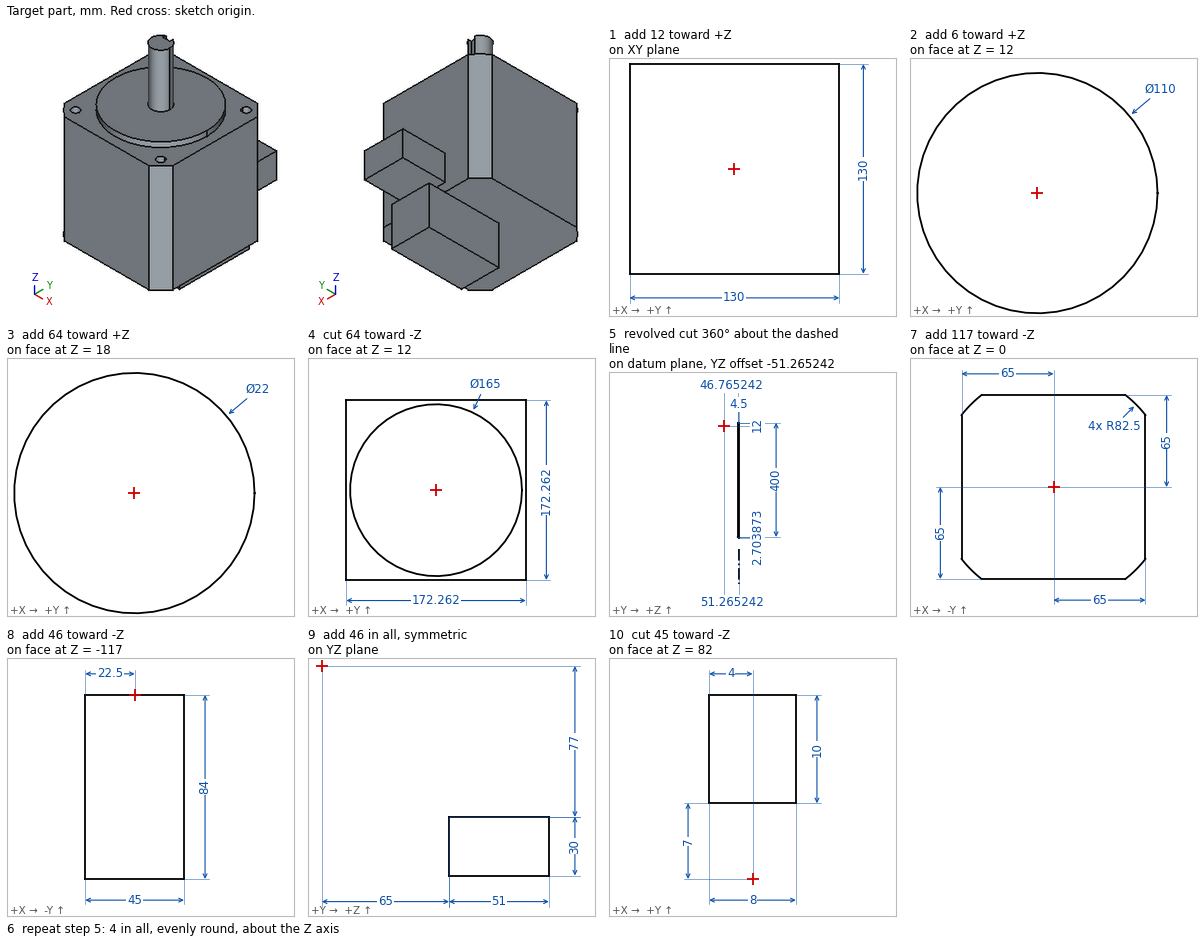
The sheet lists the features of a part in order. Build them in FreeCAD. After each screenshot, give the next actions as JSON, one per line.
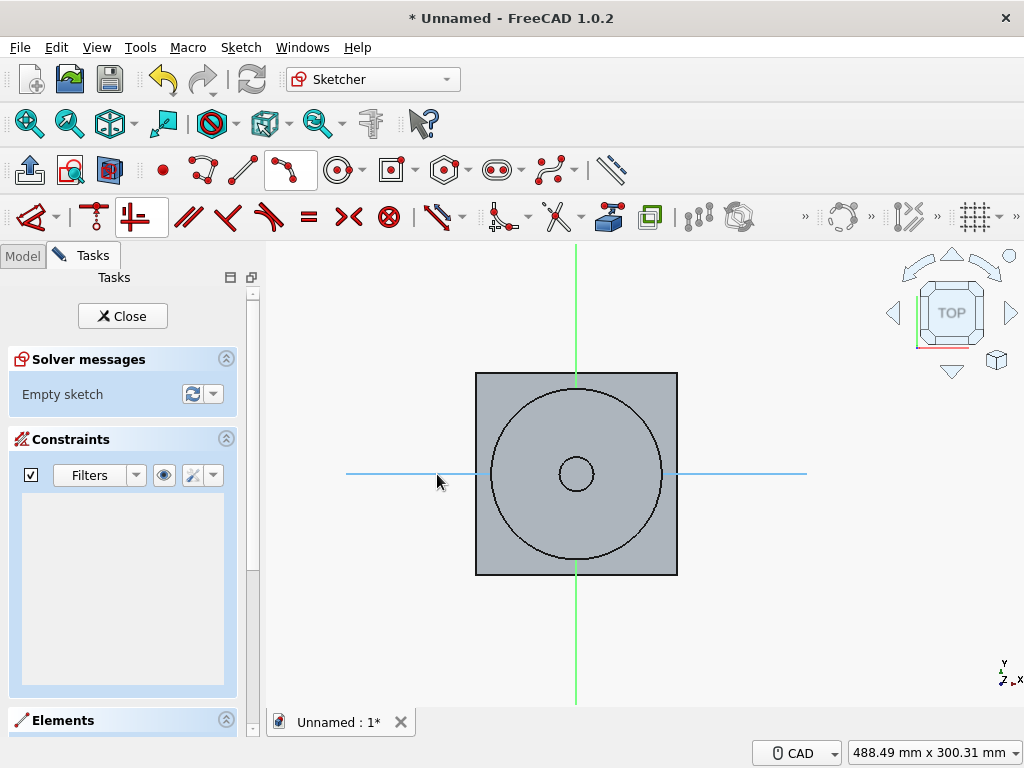
{"action": "left_click", "coordinate": [392, 170]}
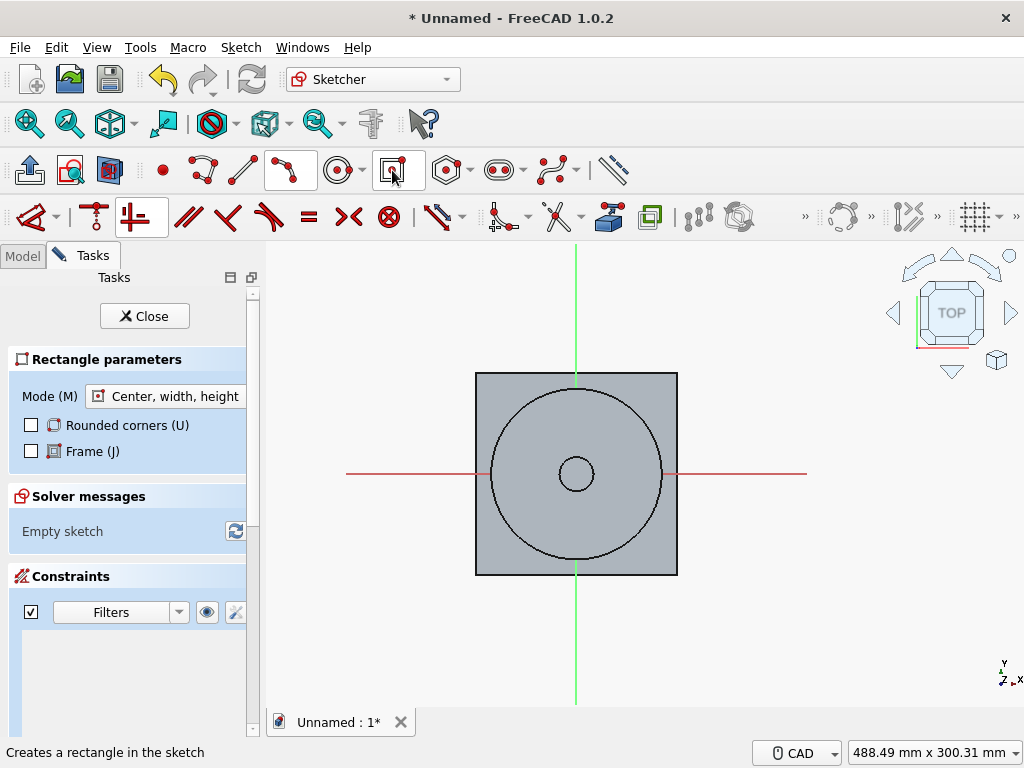
{"action": "left_click", "coordinate": [577, 474]}
{"action": "mouse_move", "coordinate": [710, 341]}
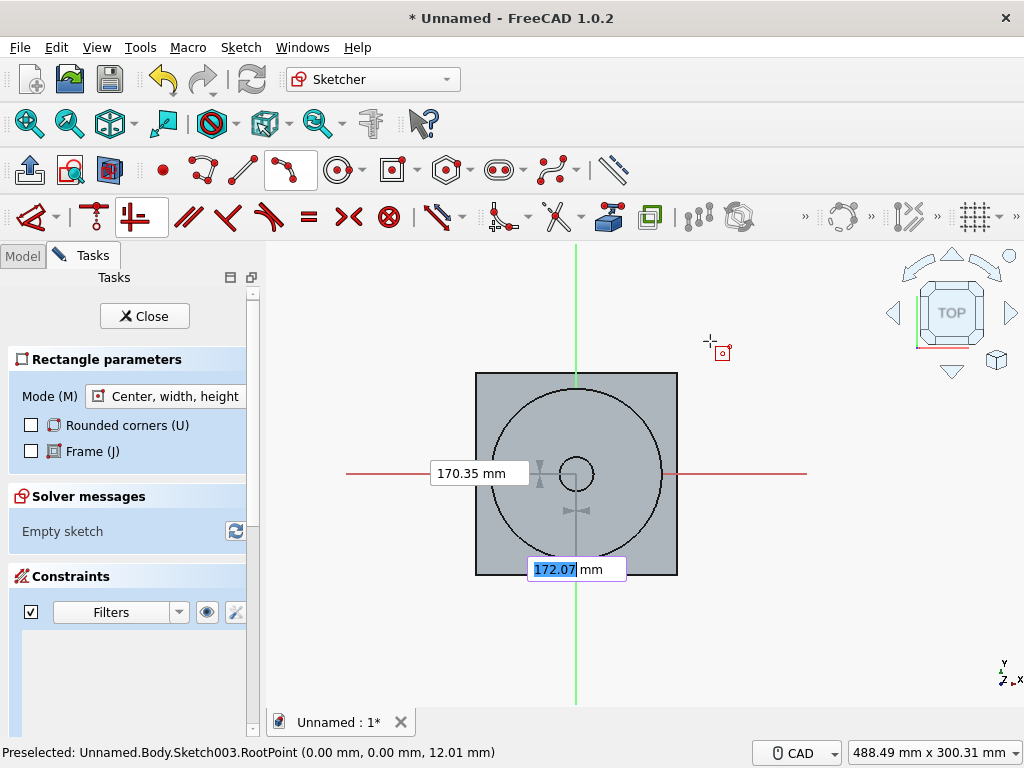
{"action": "type", "text": "172.262"}
{"action": "key", "text": "Tab"}
{"action": "type", "text": "172.262"}
{"action": "key", "text": "Return"}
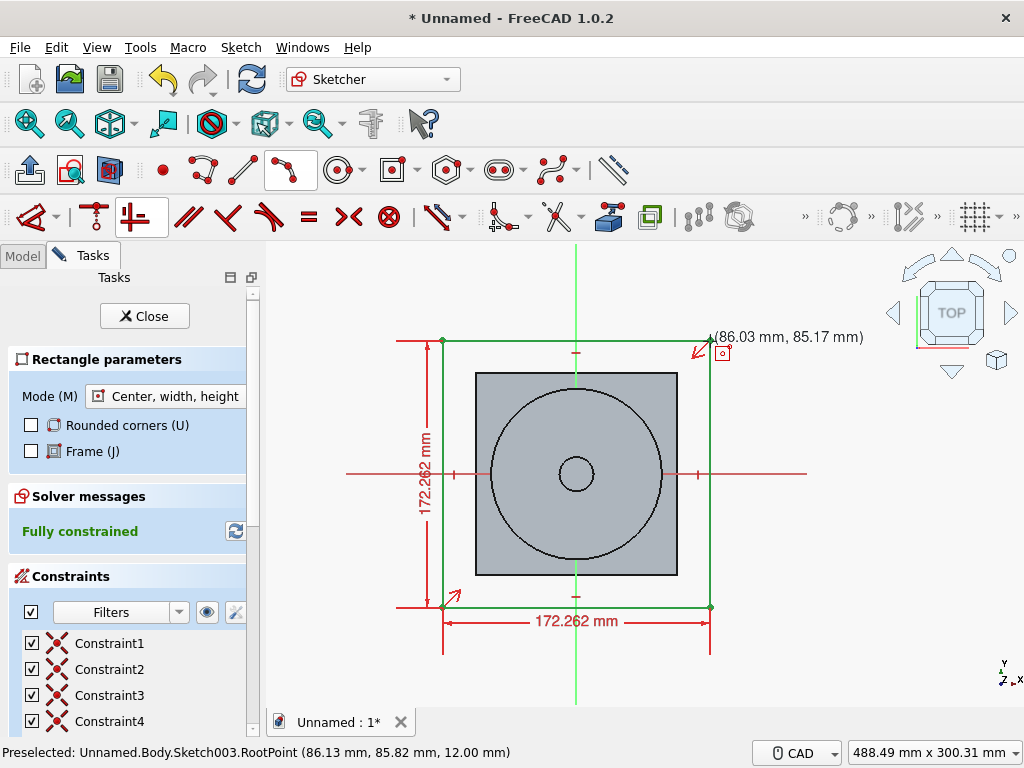
{"action": "left_click", "coordinate": [338, 170]}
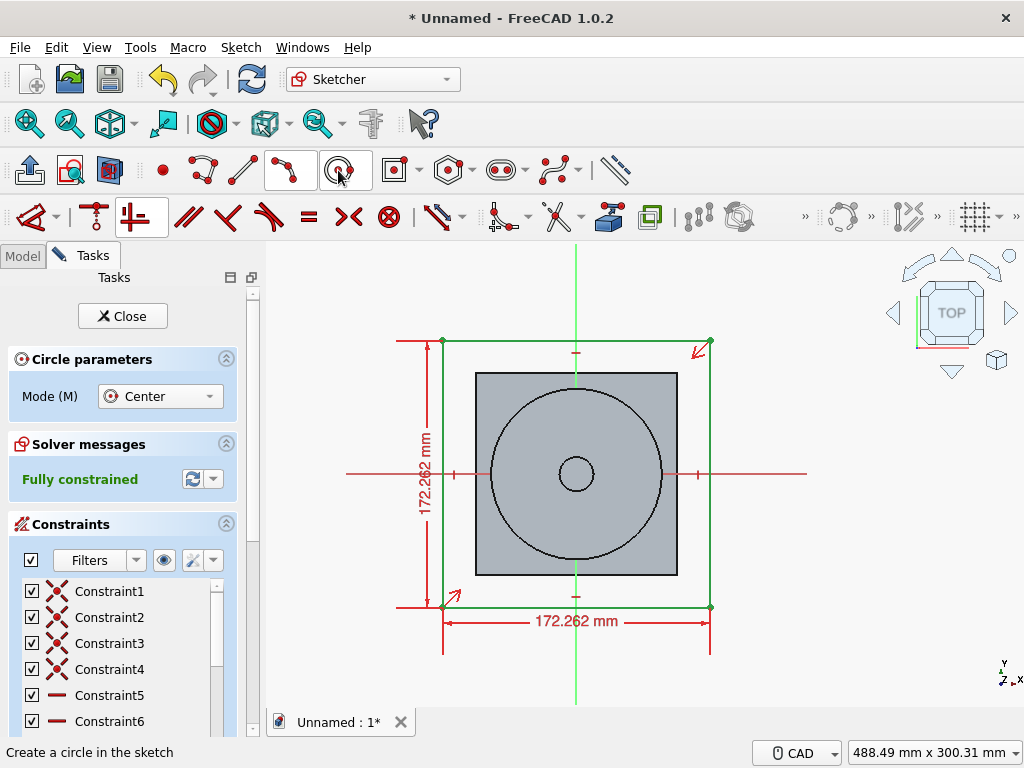
{"action": "left_click", "coordinate": [577, 474]}
{"action": "mouse_move", "coordinate": [667, 384]}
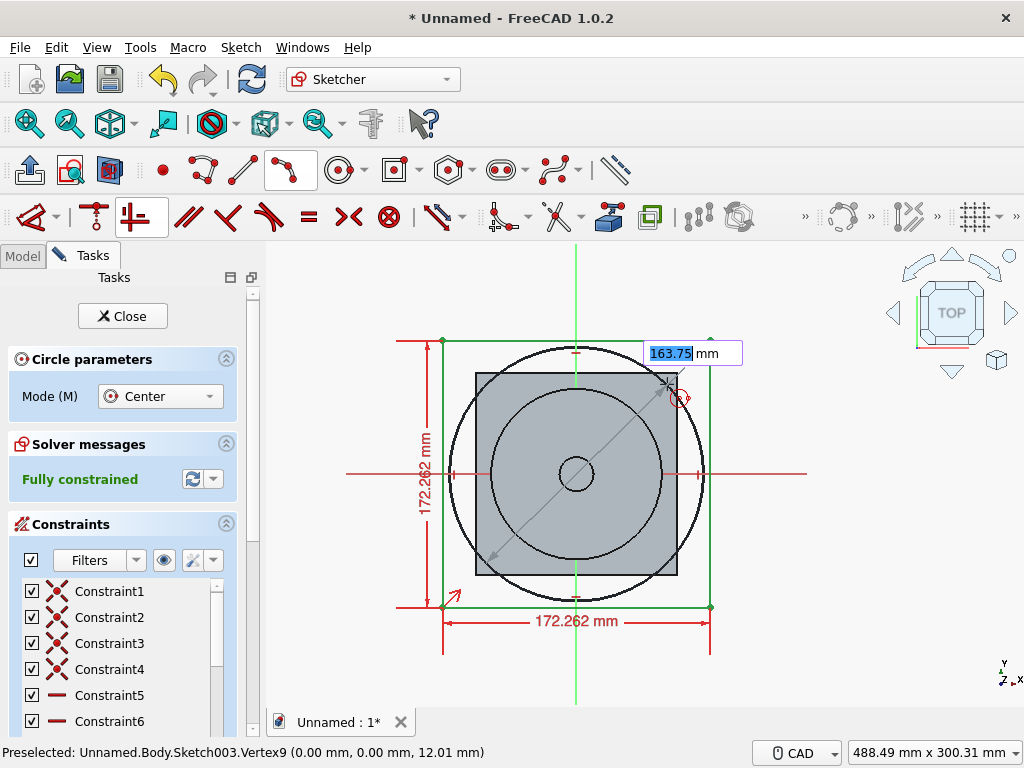
{"action": "type", "text": "165"}
{"action": "key", "text": "Return"}
{"action": "key", "text": "Escape"}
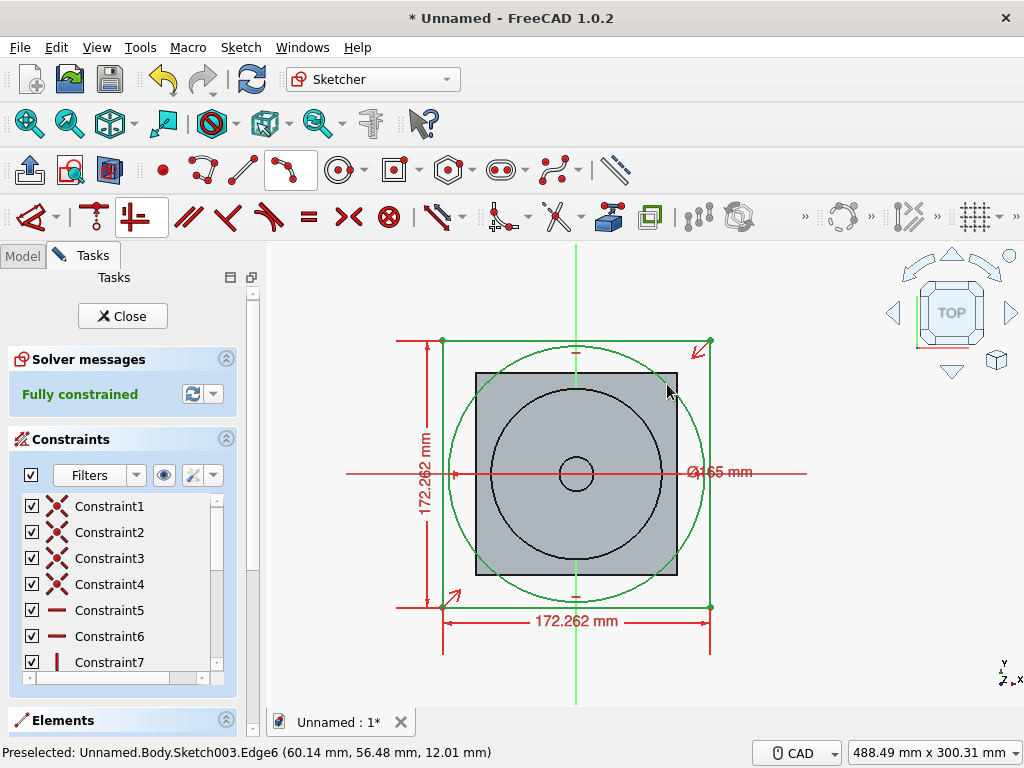
{"action": "left_click", "coordinate": [123, 316]}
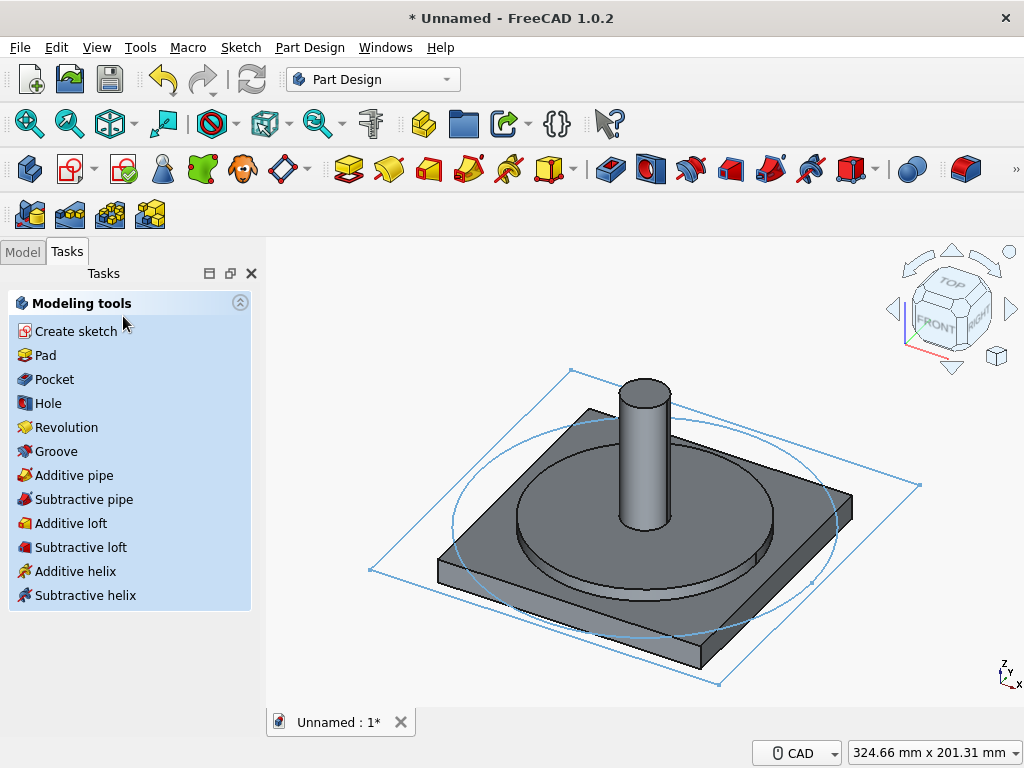
{"action": "left_click", "coordinate": [612, 170]}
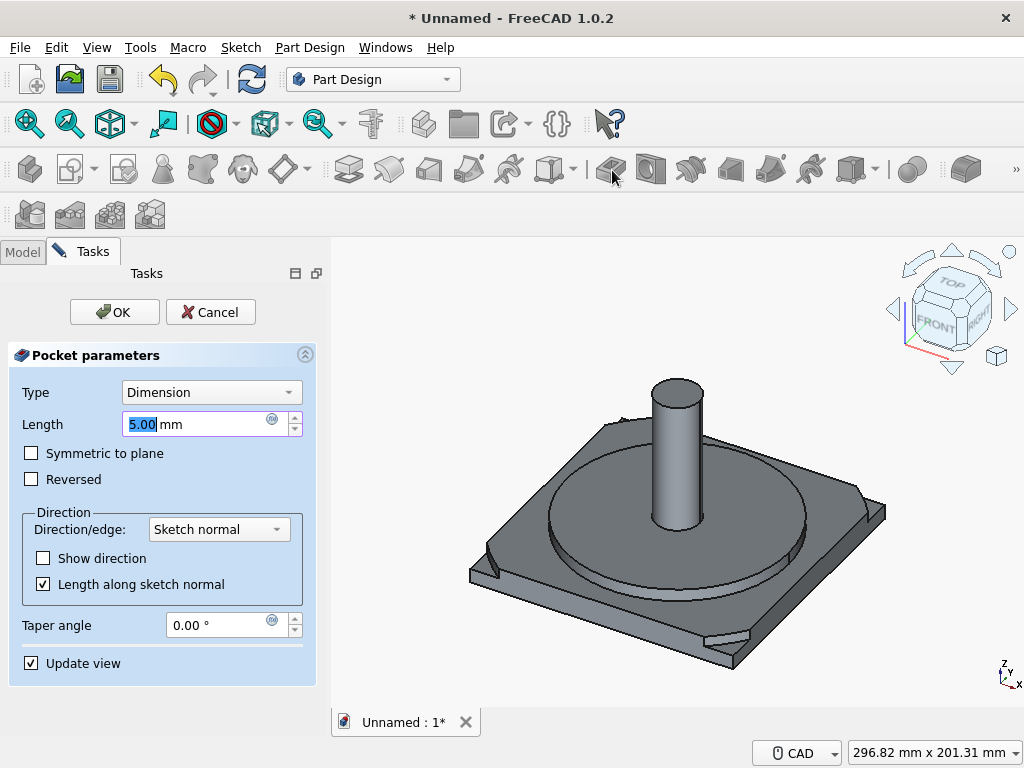
{"action": "type", "text": "64"}
{"action": "key", "text": "Tab"}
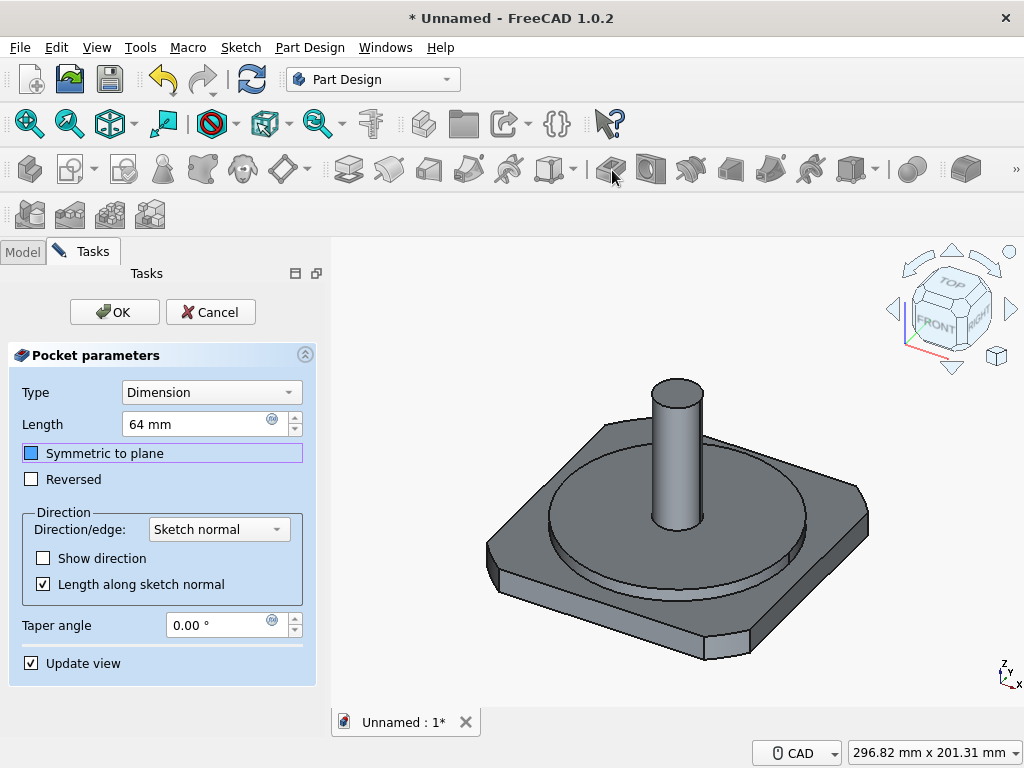
{"action": "left_click", "coordinate": [115, 312]}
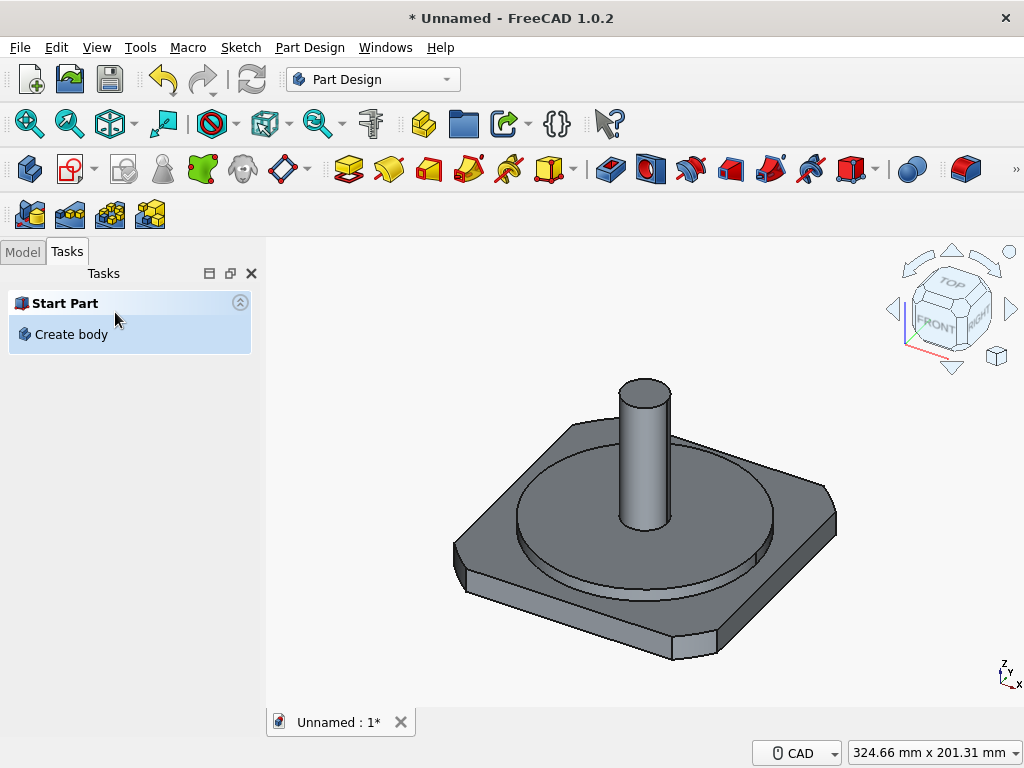
{"action": "left_click", "coordinate": [23, 251]}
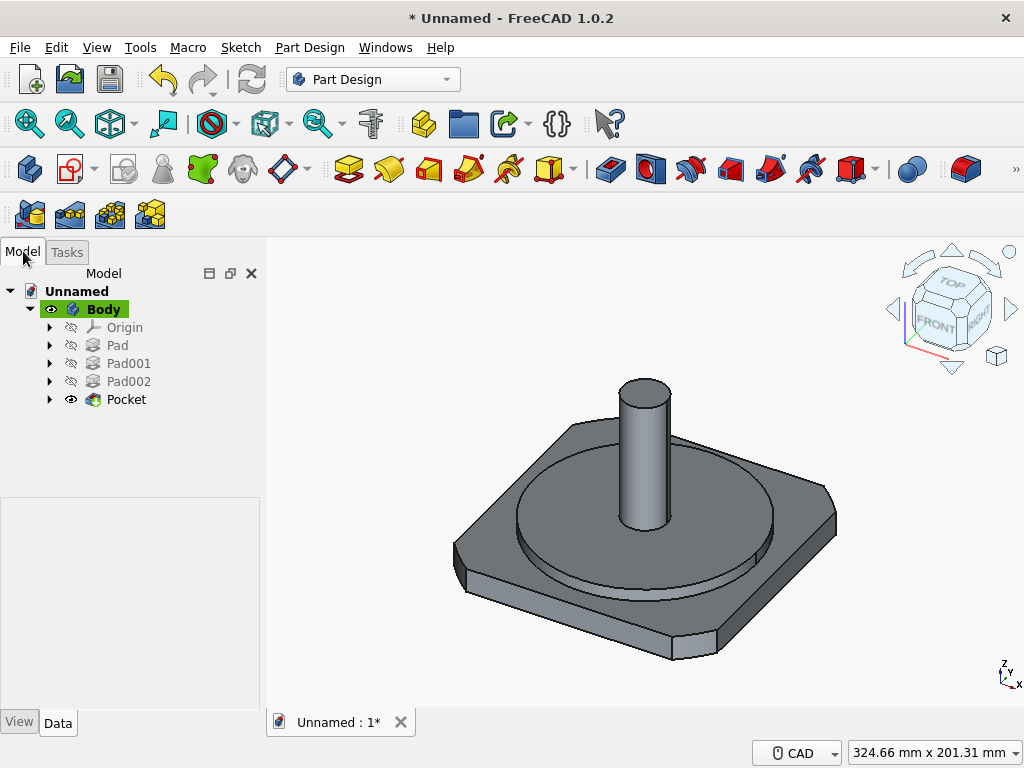
{"action": "left_click", "coordinate": [50, 327]}